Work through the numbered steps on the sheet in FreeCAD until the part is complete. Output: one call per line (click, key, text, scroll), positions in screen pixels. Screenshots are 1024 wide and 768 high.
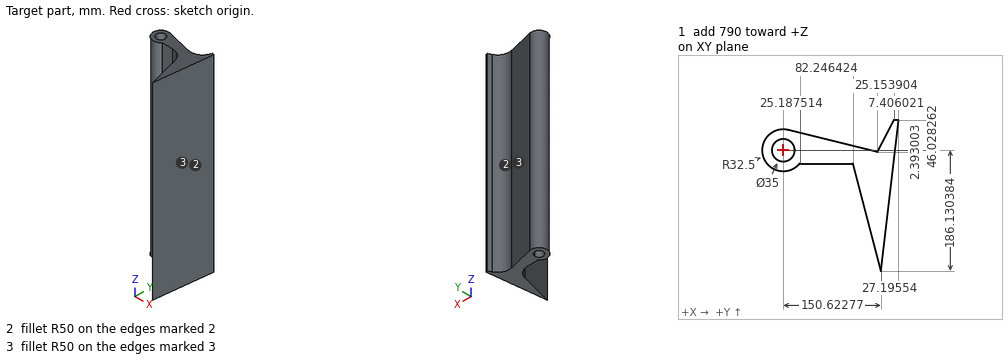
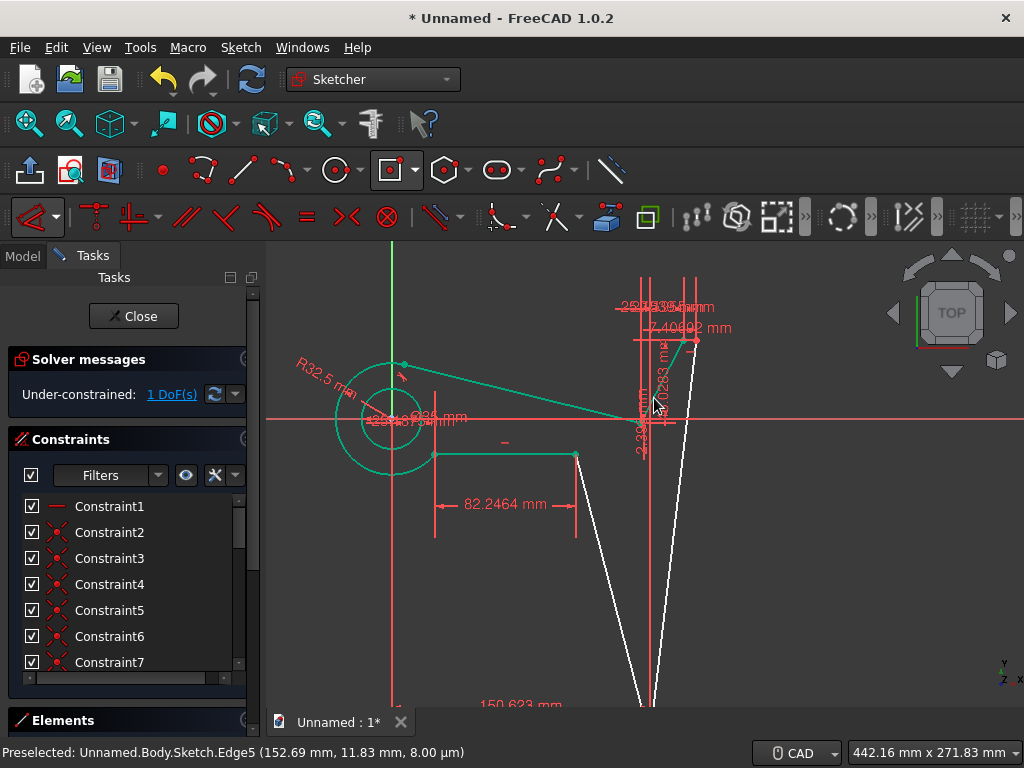
scroll(696, 342, down, 2)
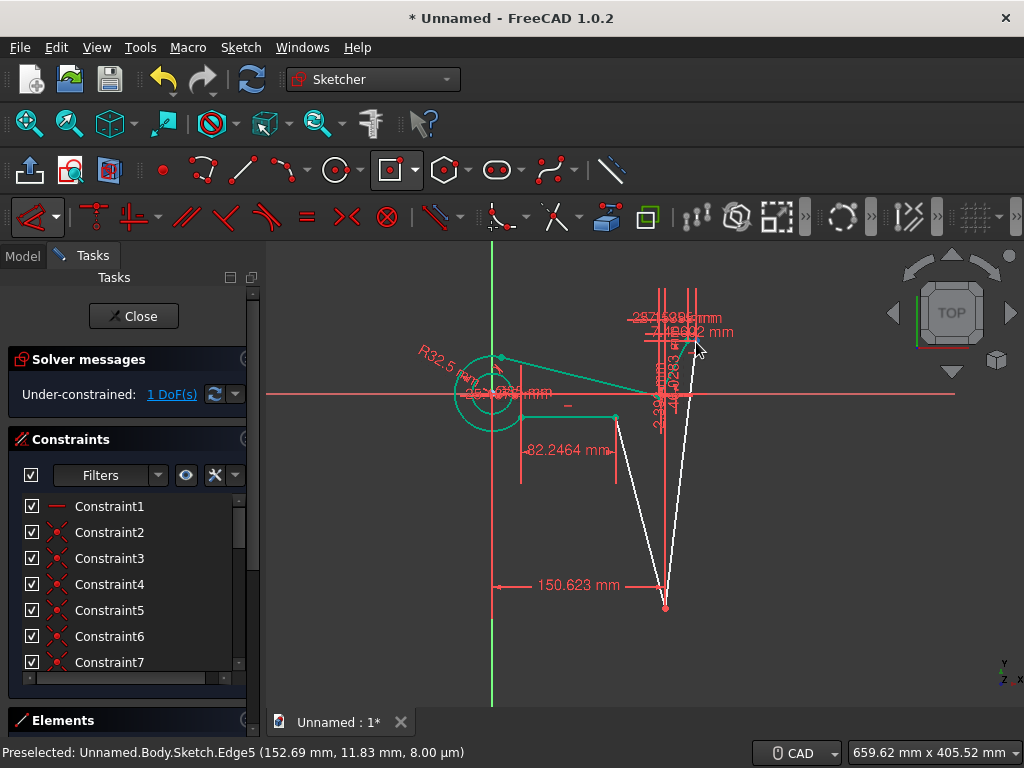
click(665, 608)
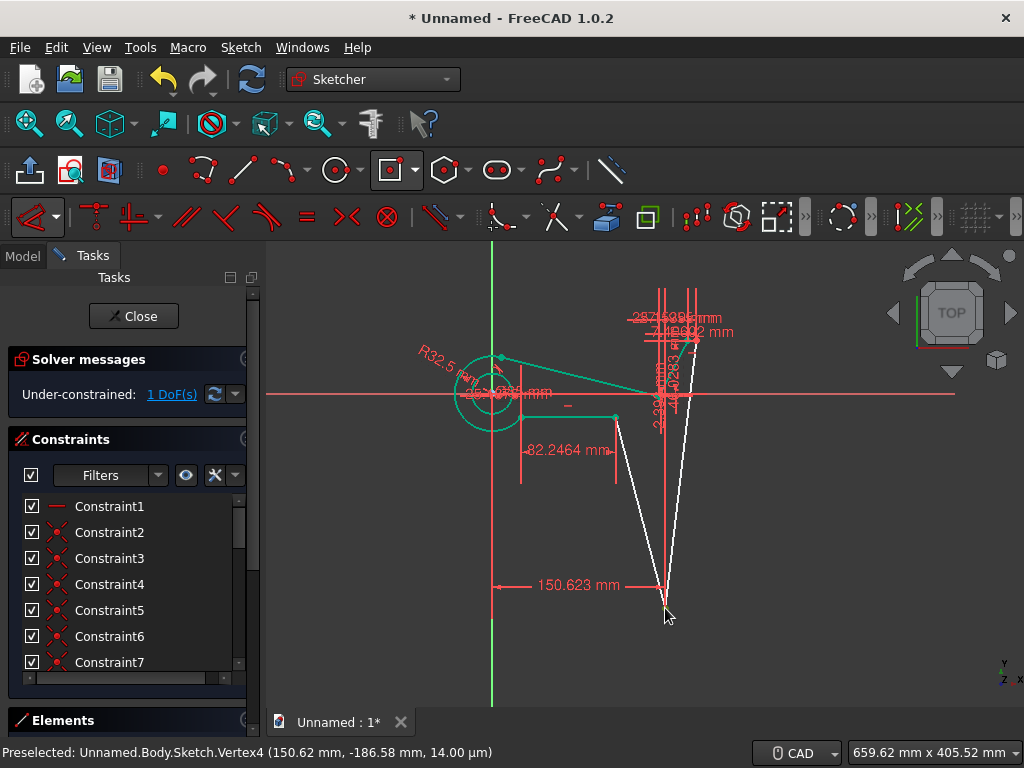
click(58, 218)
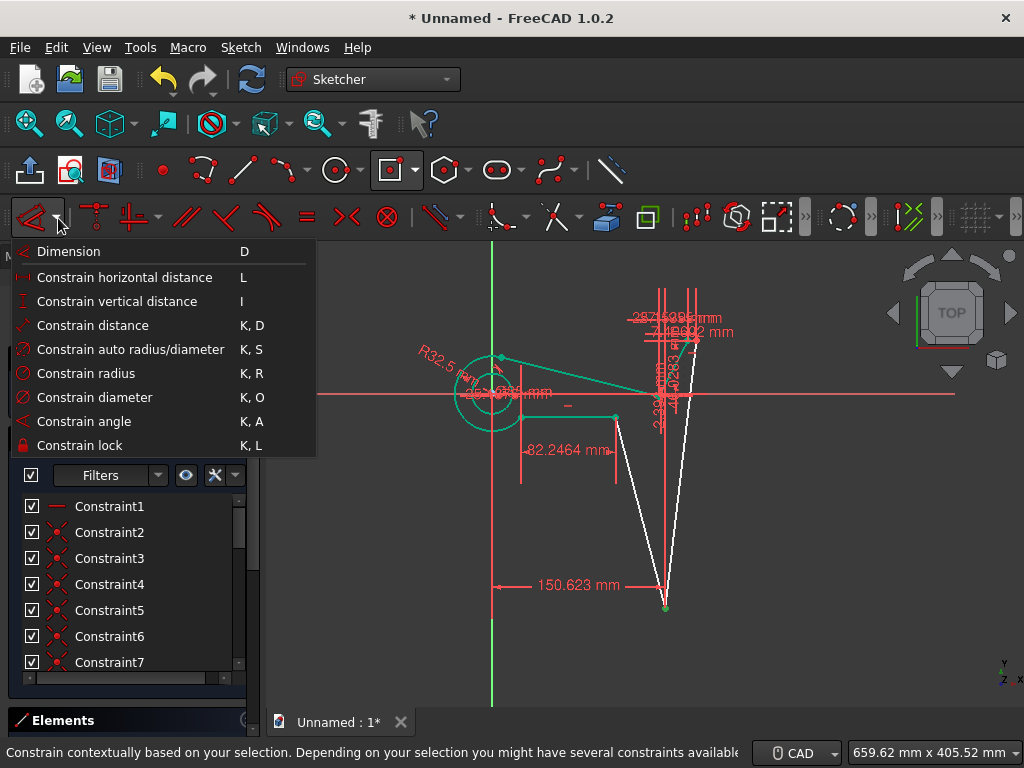
click(164, 301)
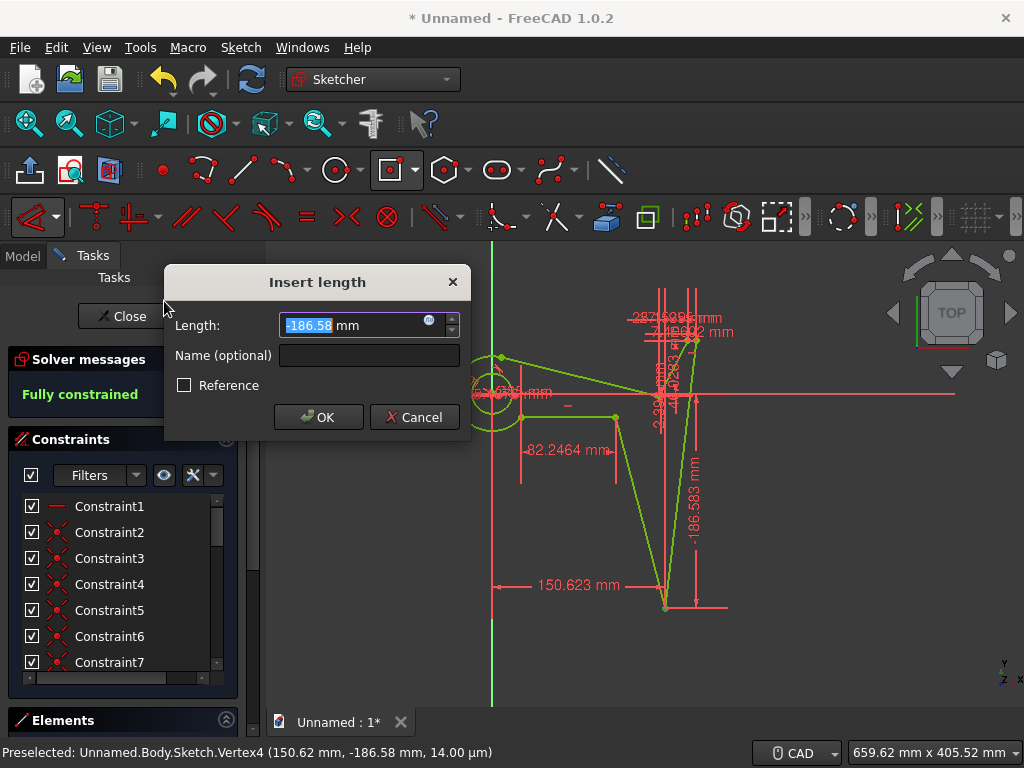
text(-186.130384)
key(Return)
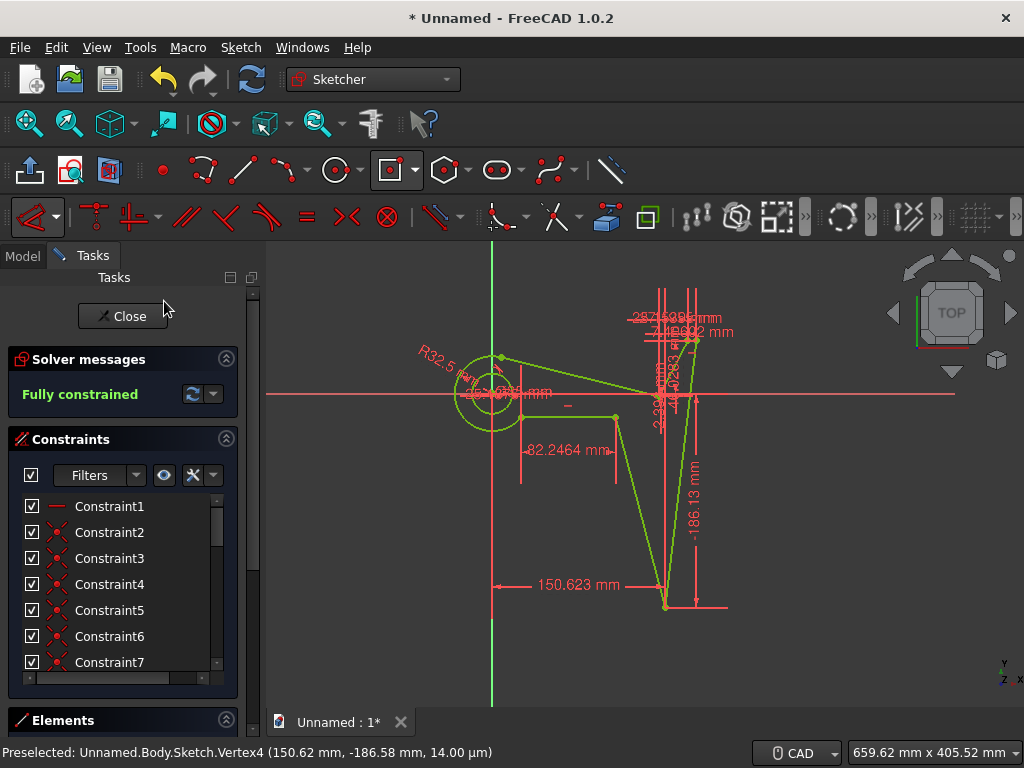
click(123, 316)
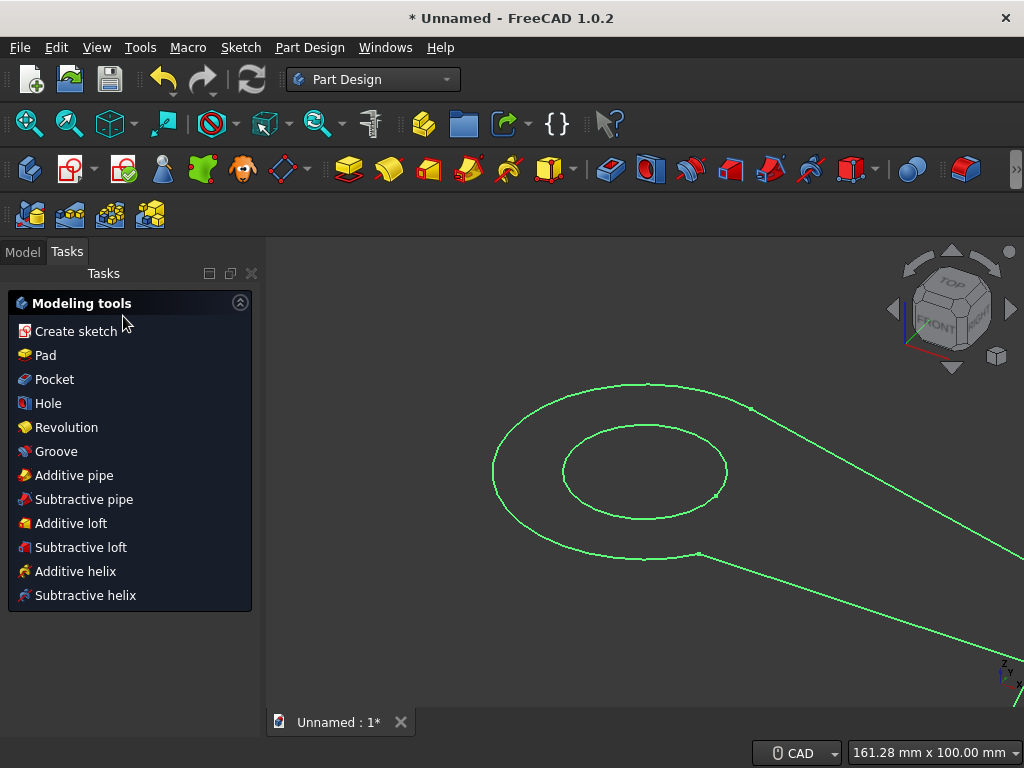
click(350, 170)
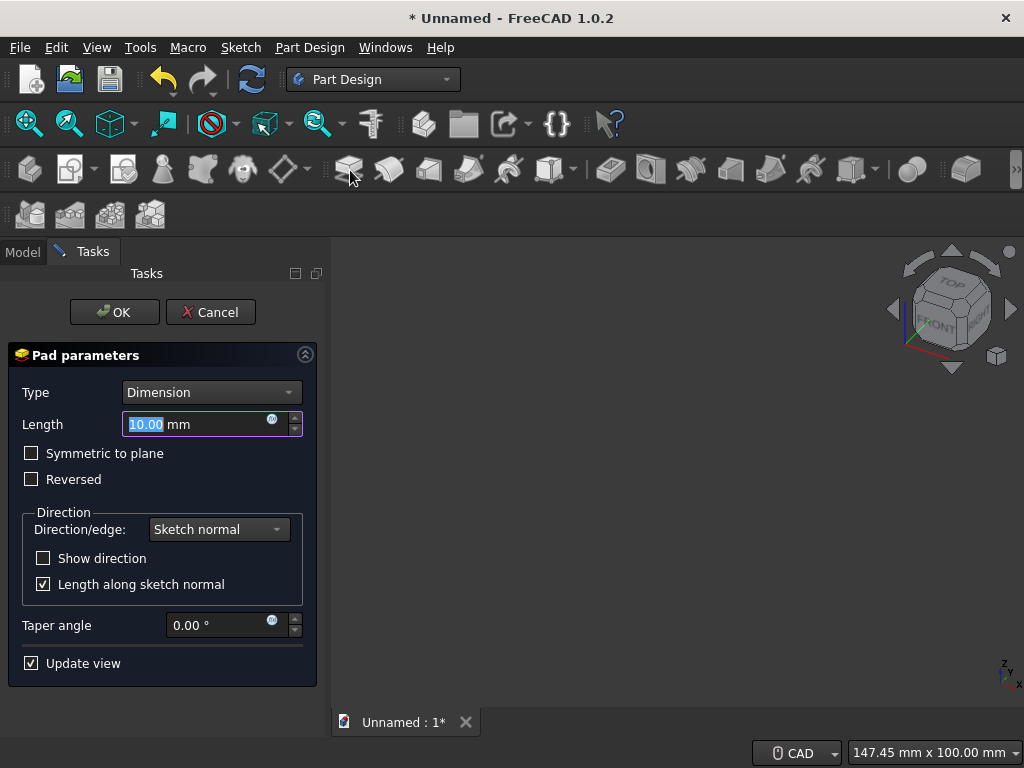
text(790)
key(Tab)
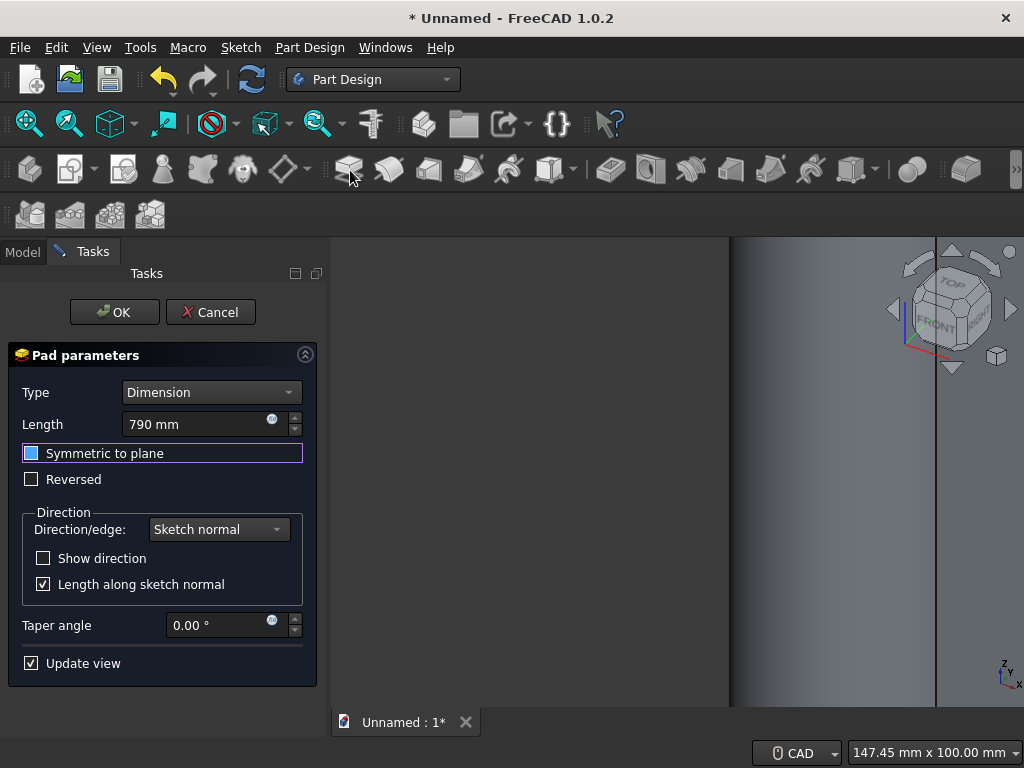
click(115, 312)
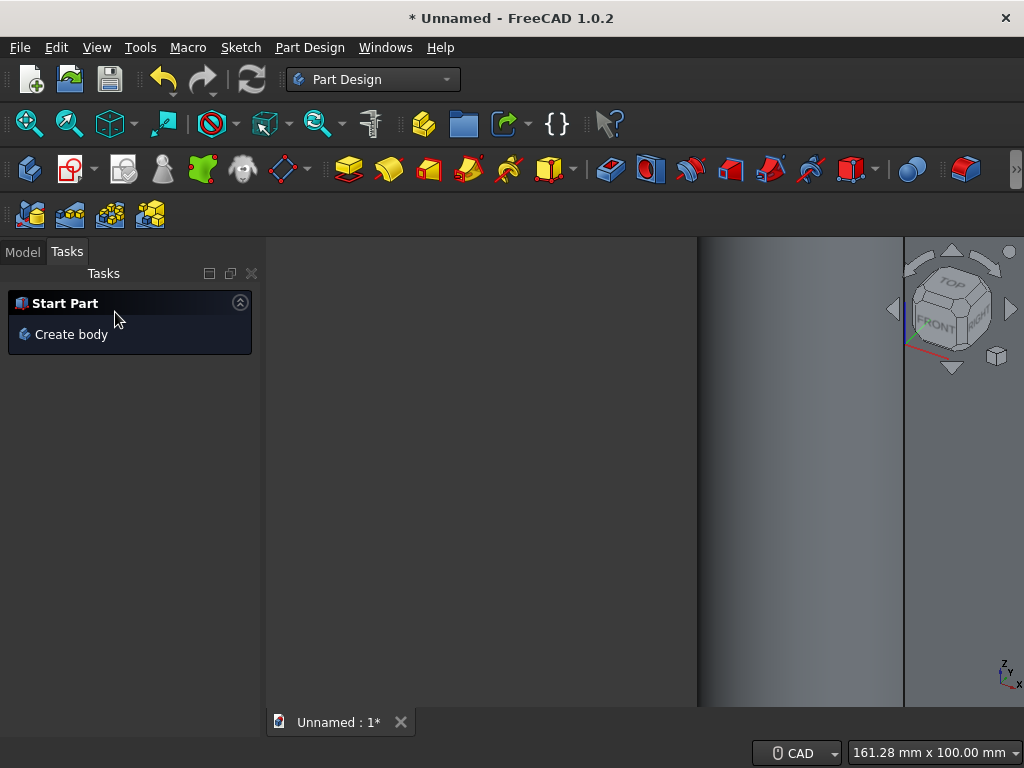
key(v)
key(f)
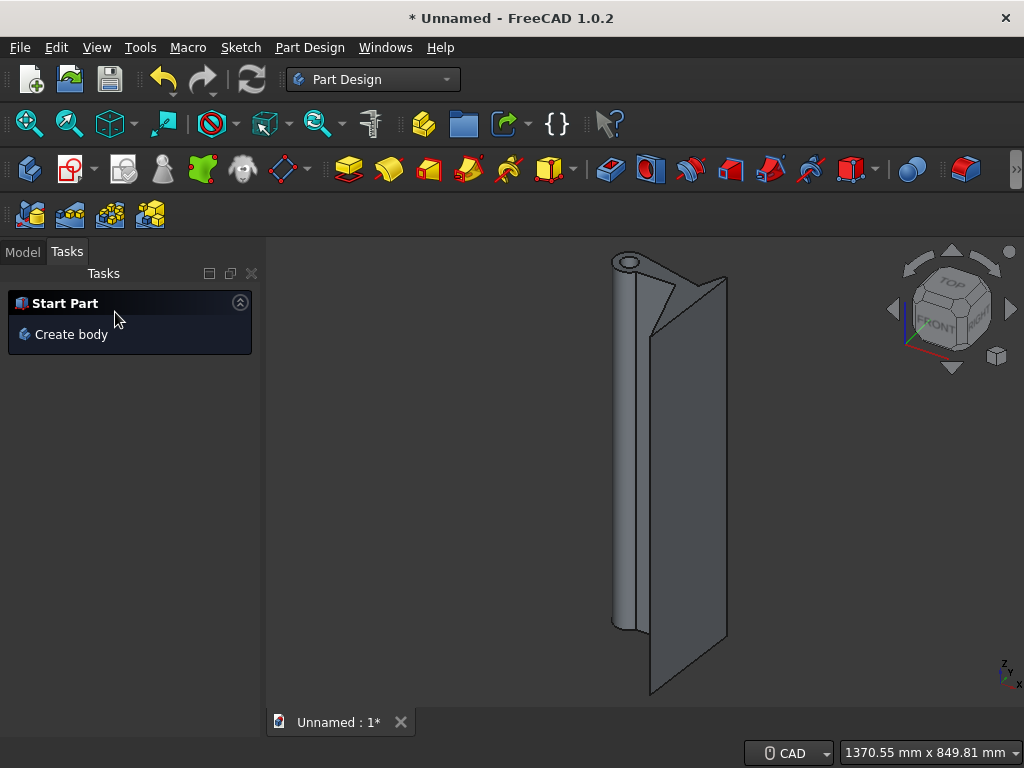
key(0)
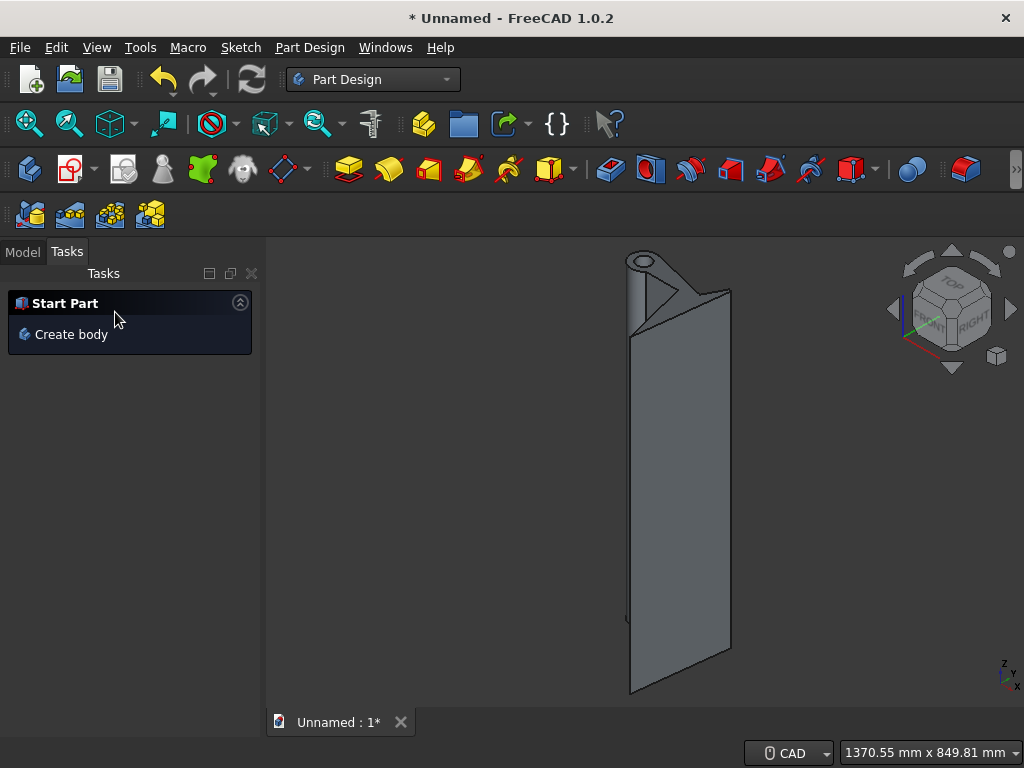
key(2)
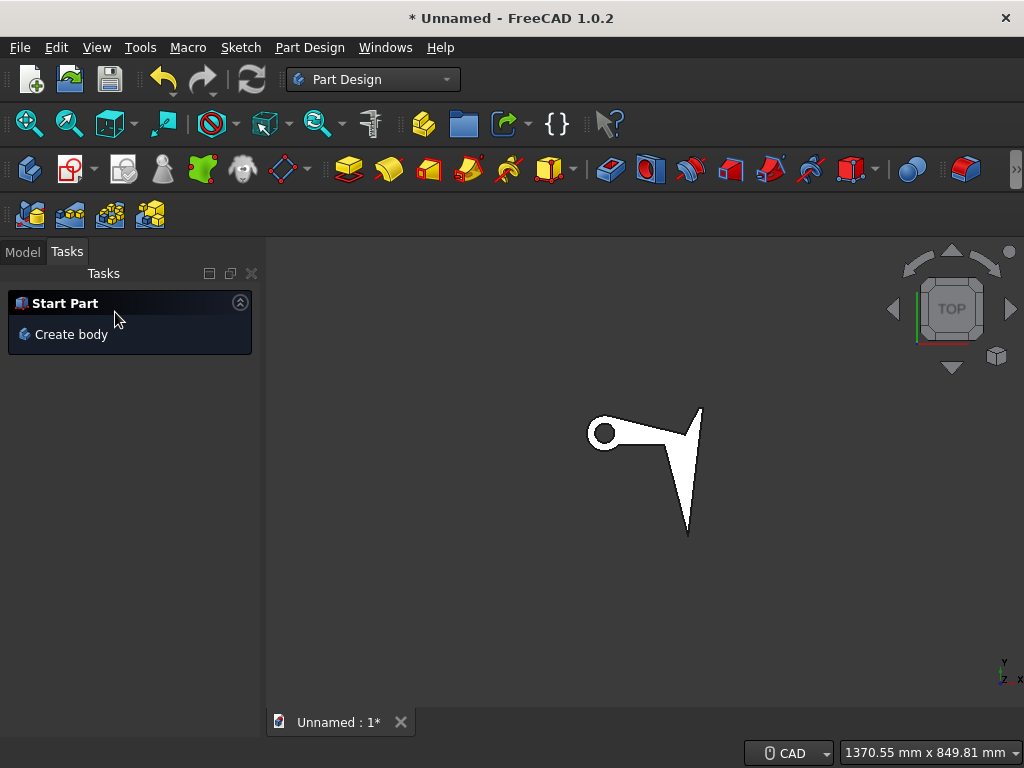
click(30, 124)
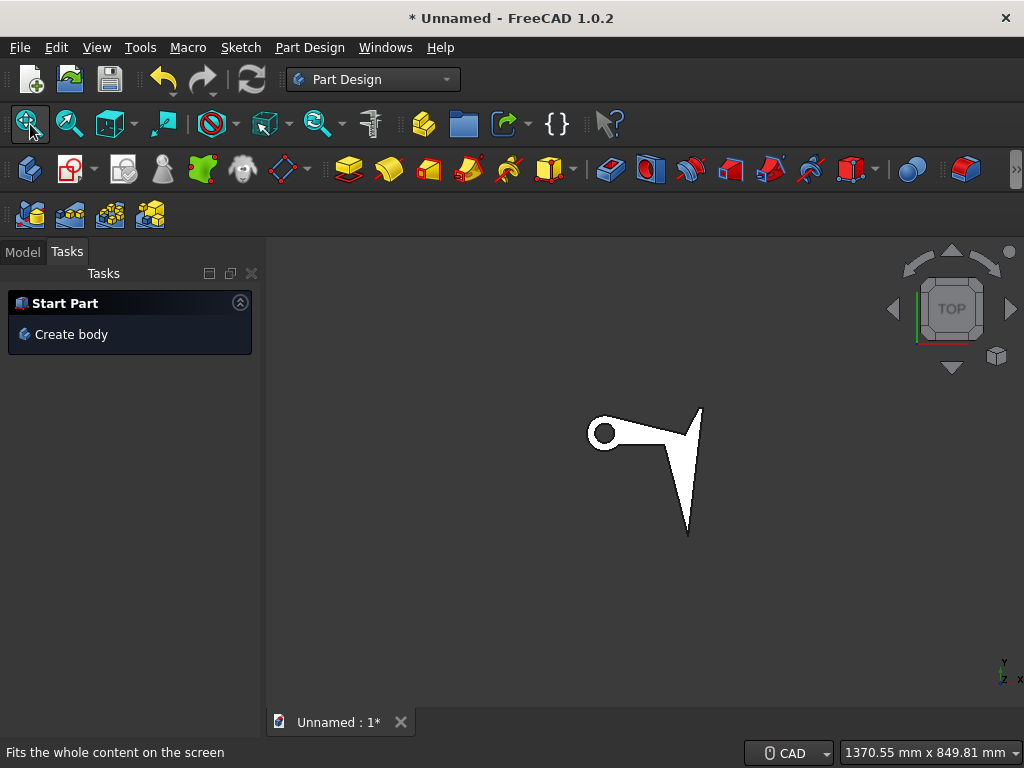
key(1)